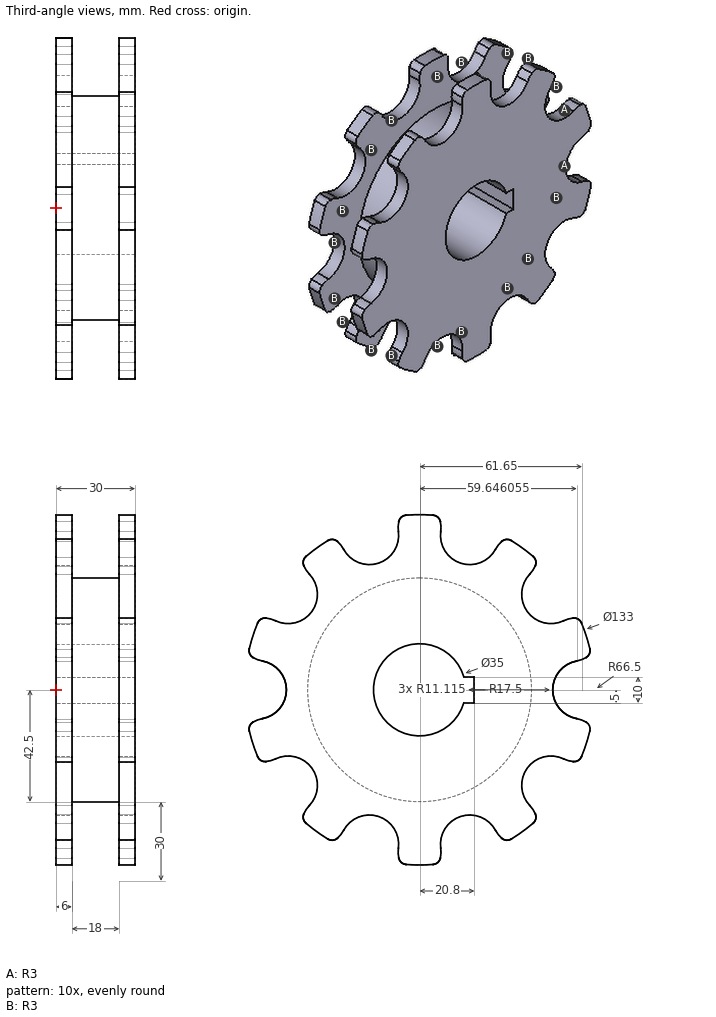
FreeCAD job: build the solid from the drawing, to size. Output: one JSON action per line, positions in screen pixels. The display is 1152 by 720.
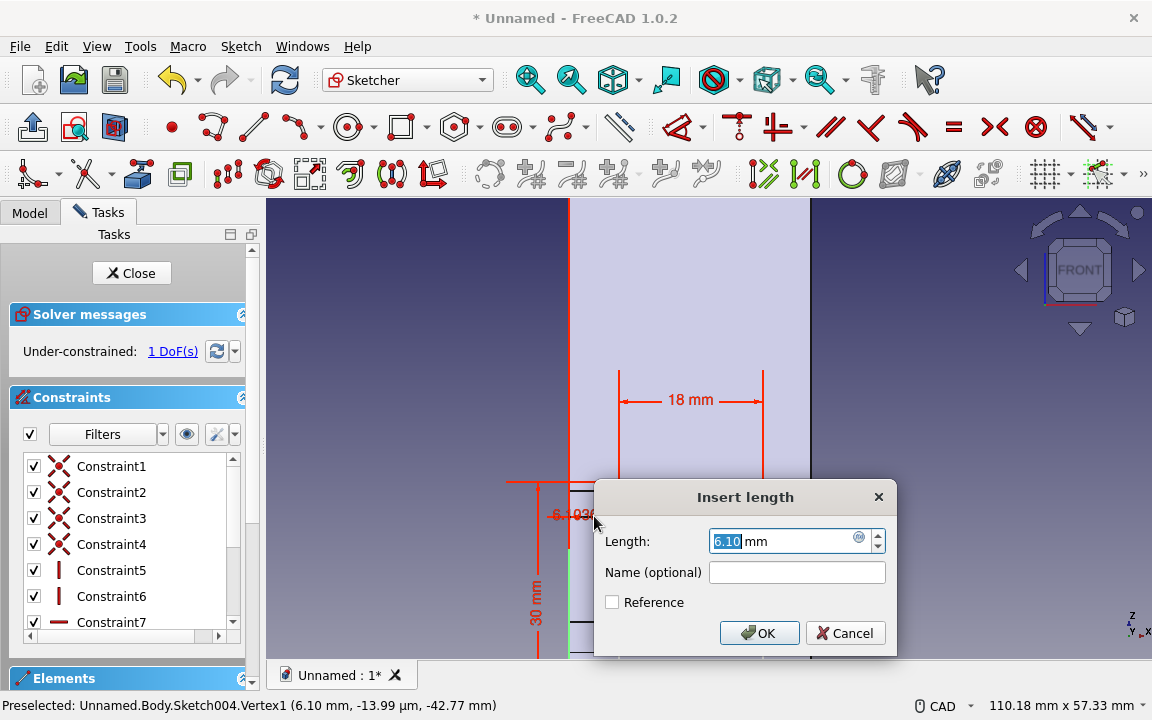
{"action": "type", "text": "6"}
{"action": "key", "text": "Return"}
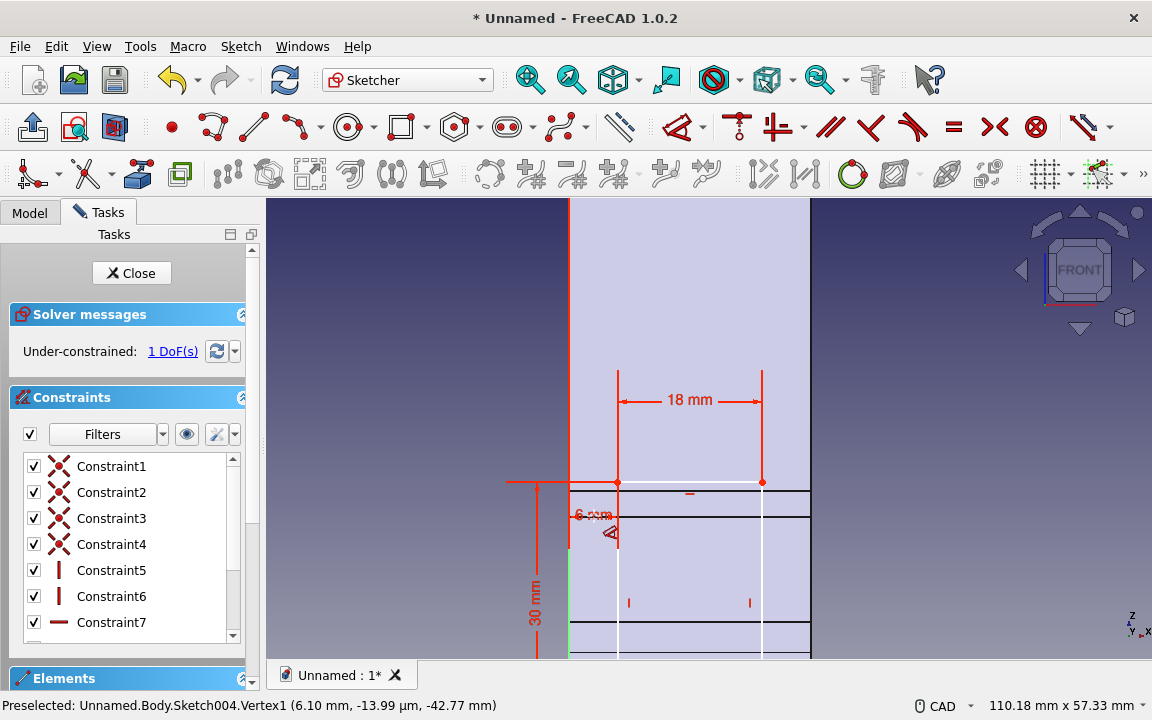
{"action": "left_click", "coordinate": [618, 482]}
{"action": "left_click", "coordinate": [535, 354]}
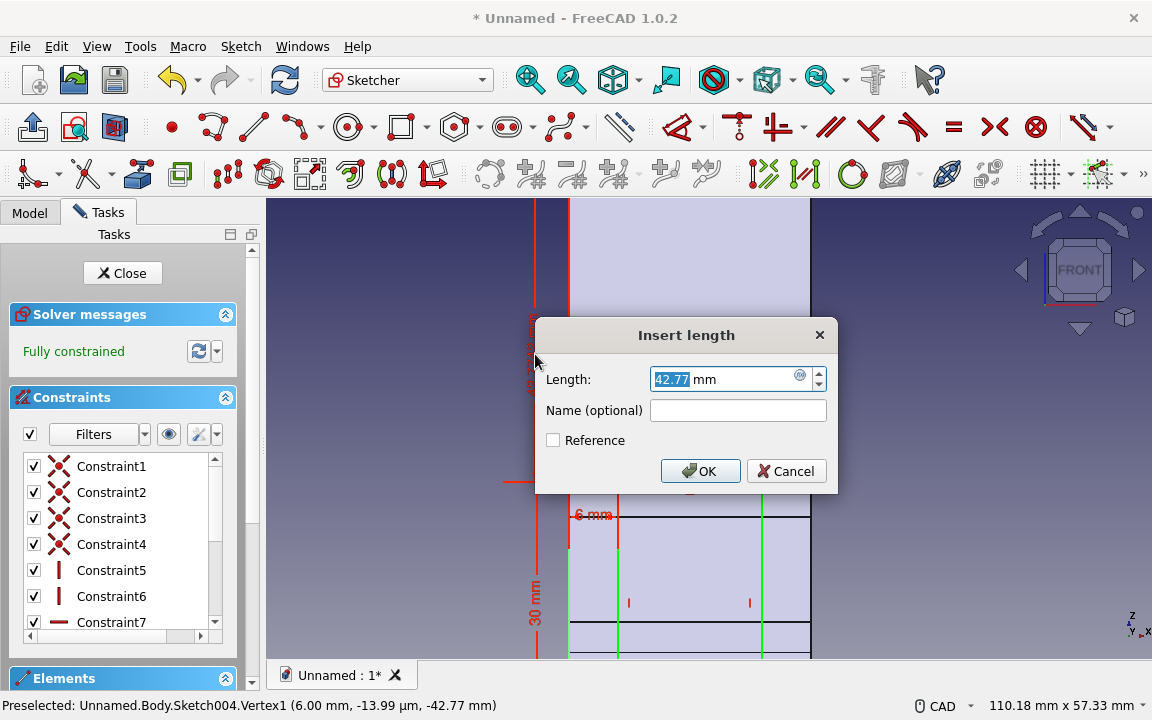
{"action": "type", "text": "42.5"}
{"action": "key", "text": "Return"}
{"action": "key", "text": "Escape"}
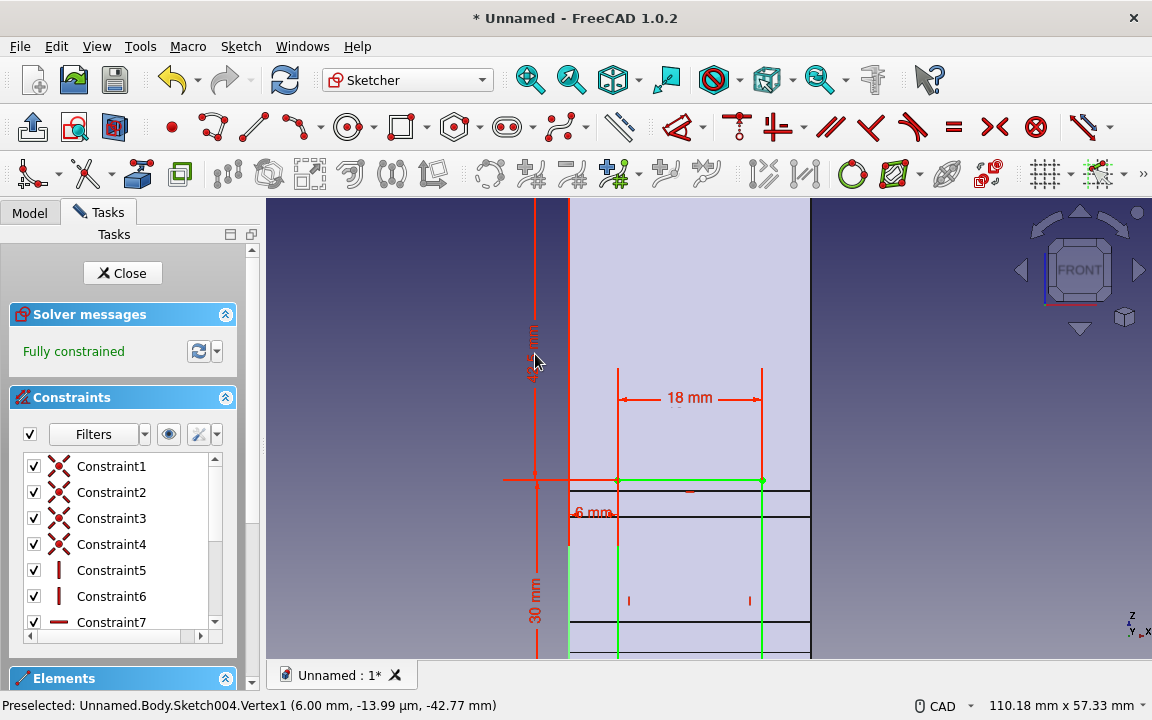
{"action": "left_click", "coordinate": [123, 273]}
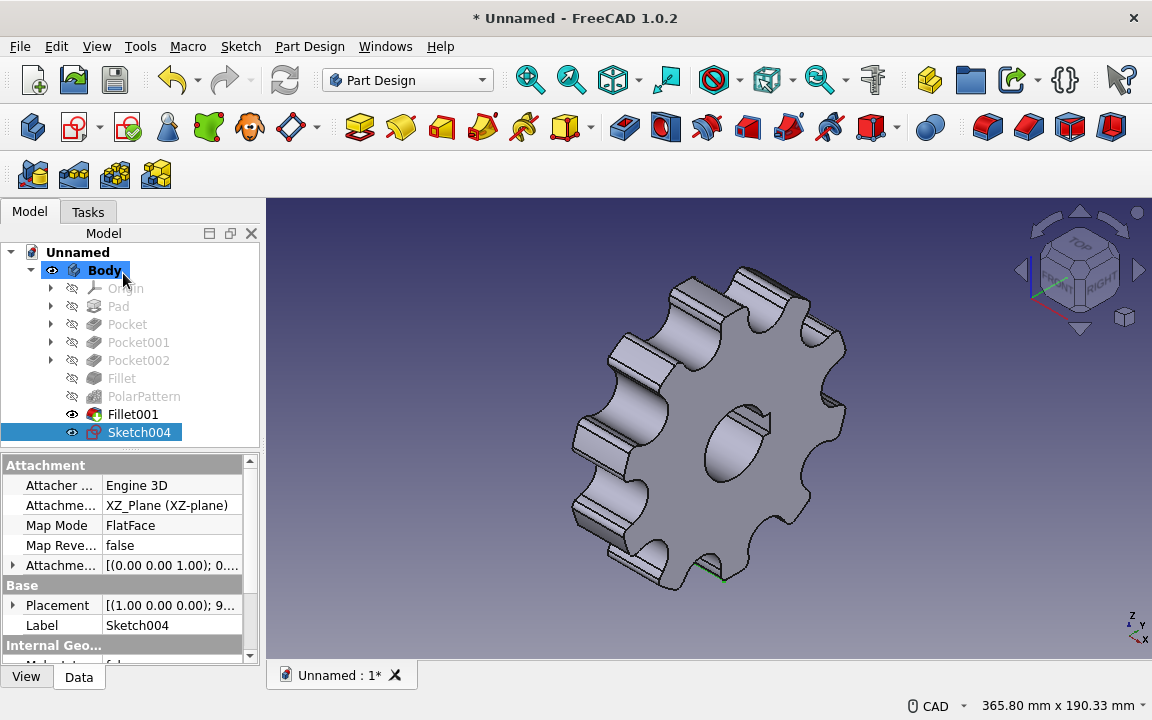
{"action": "left_click", "coordinate": [707, 128]}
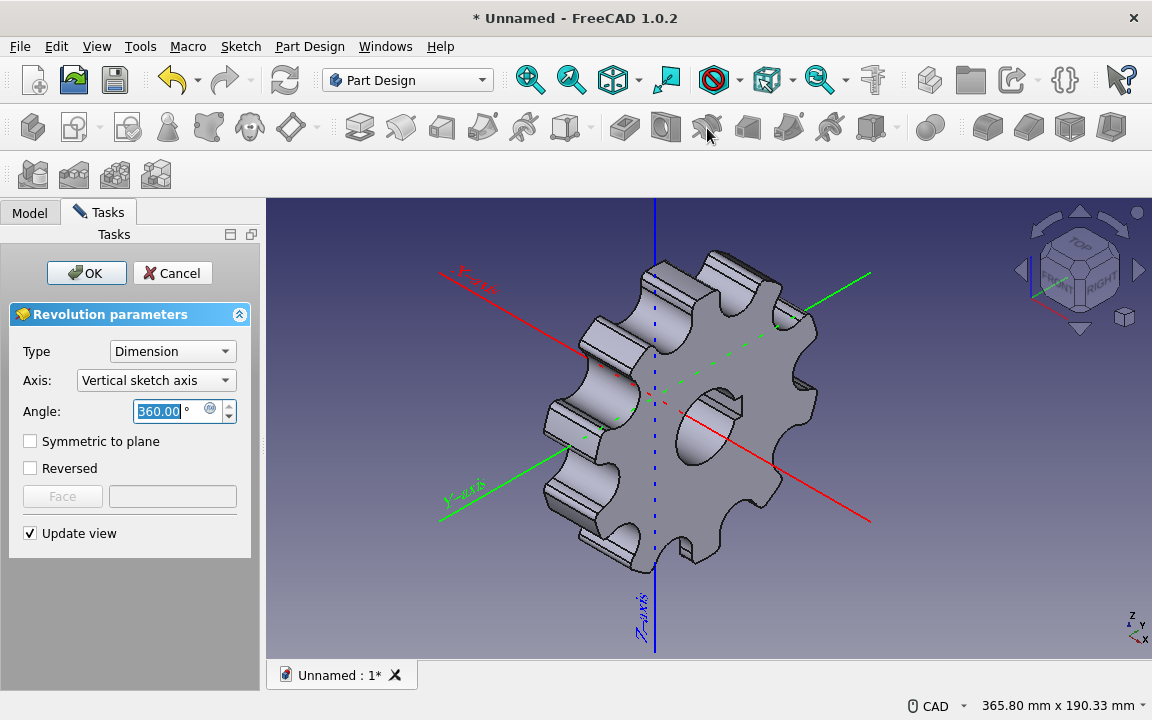
{"action": "left_click", "coordinate": [157, 380]}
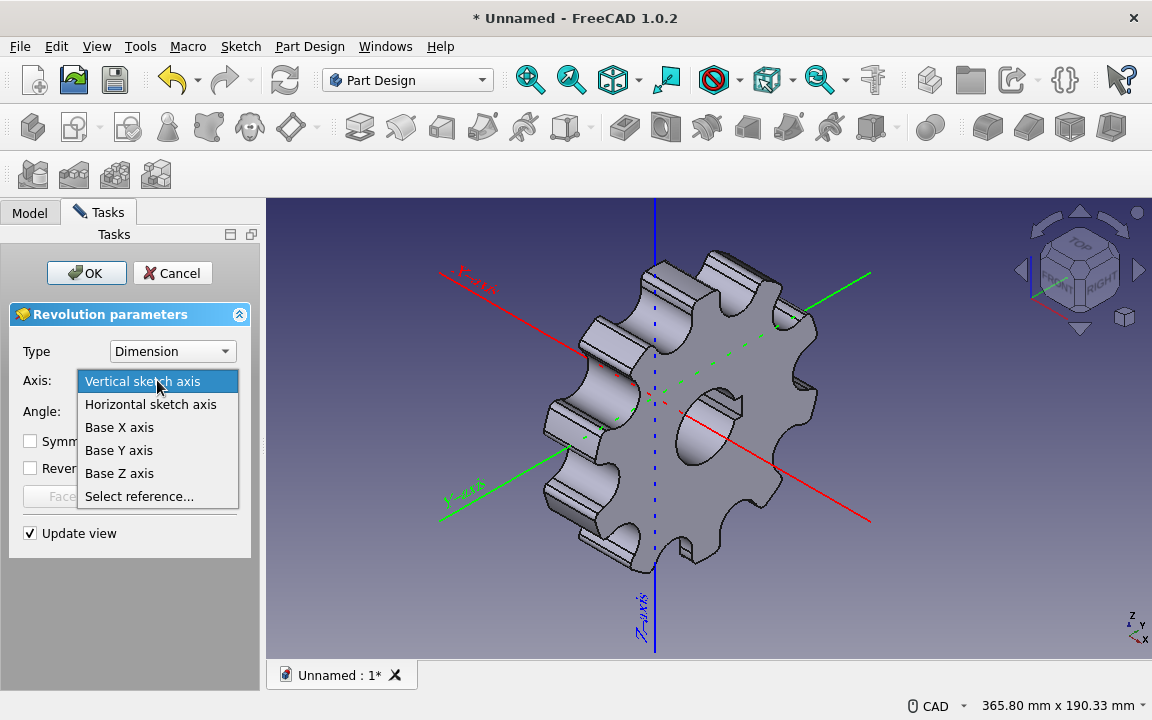
{"action": "left_click", "coordinate": [156, 404]}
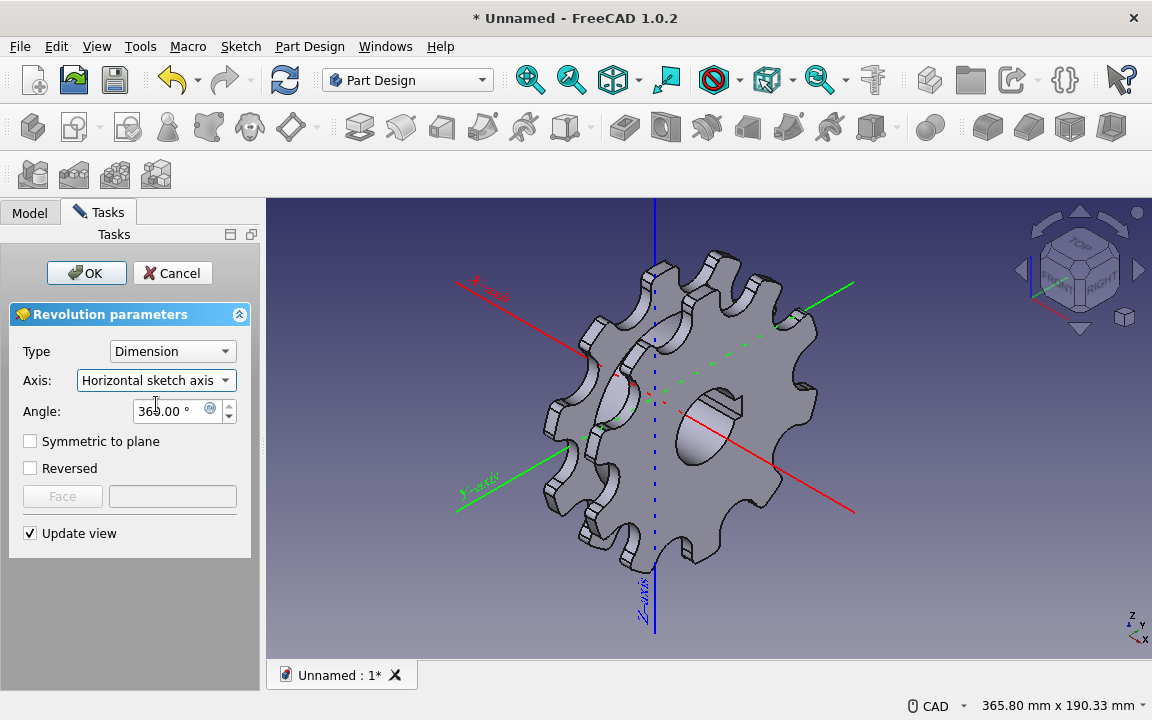
{"action": "left_click", "coordinate": [87, 273]}